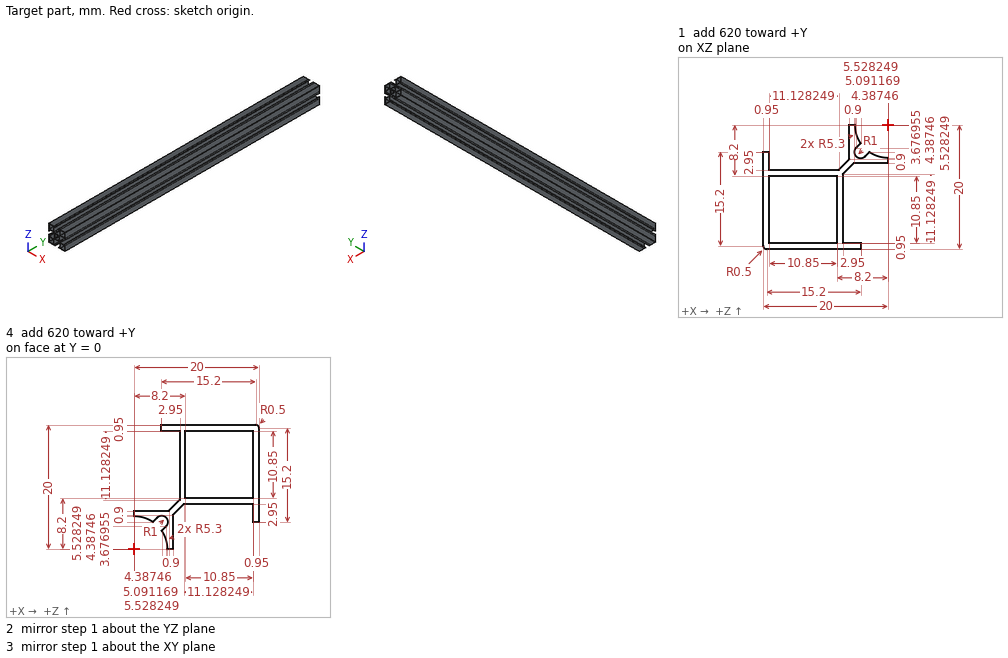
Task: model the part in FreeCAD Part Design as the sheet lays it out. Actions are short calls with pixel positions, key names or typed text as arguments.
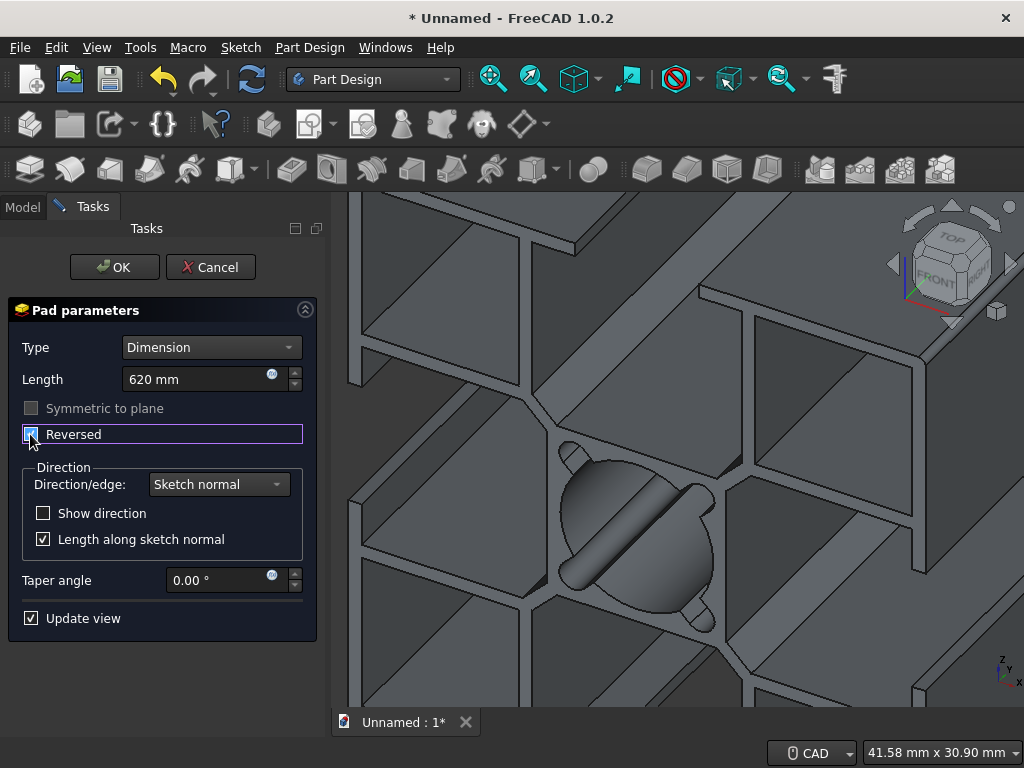
click(115, 267)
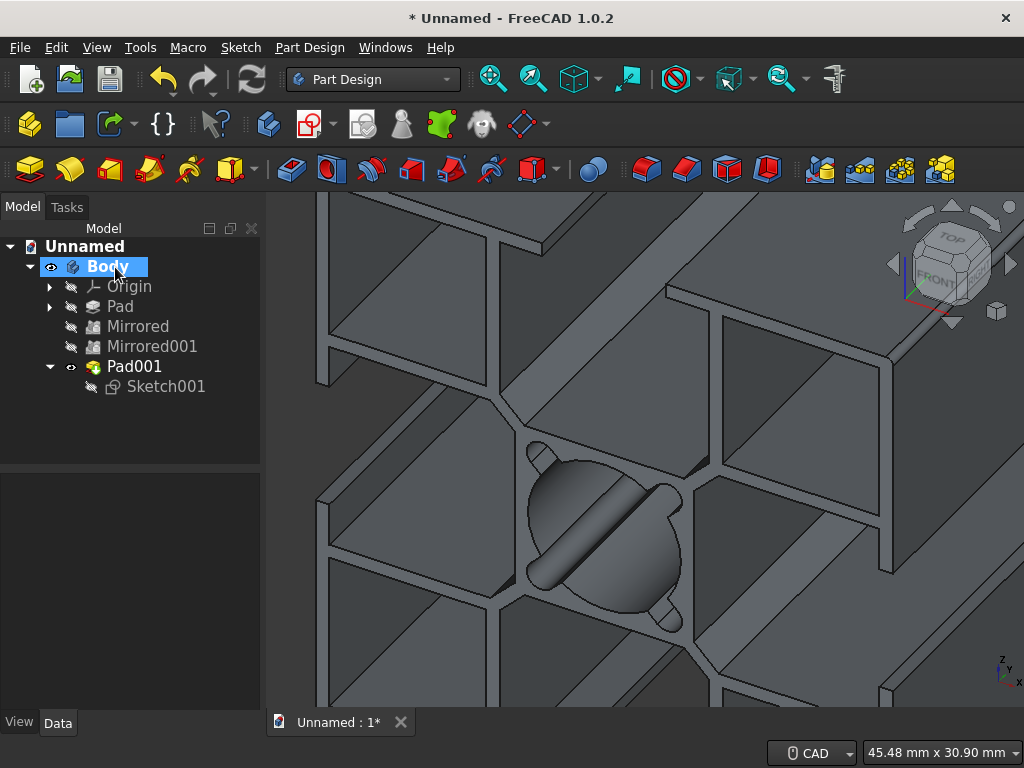
key(0)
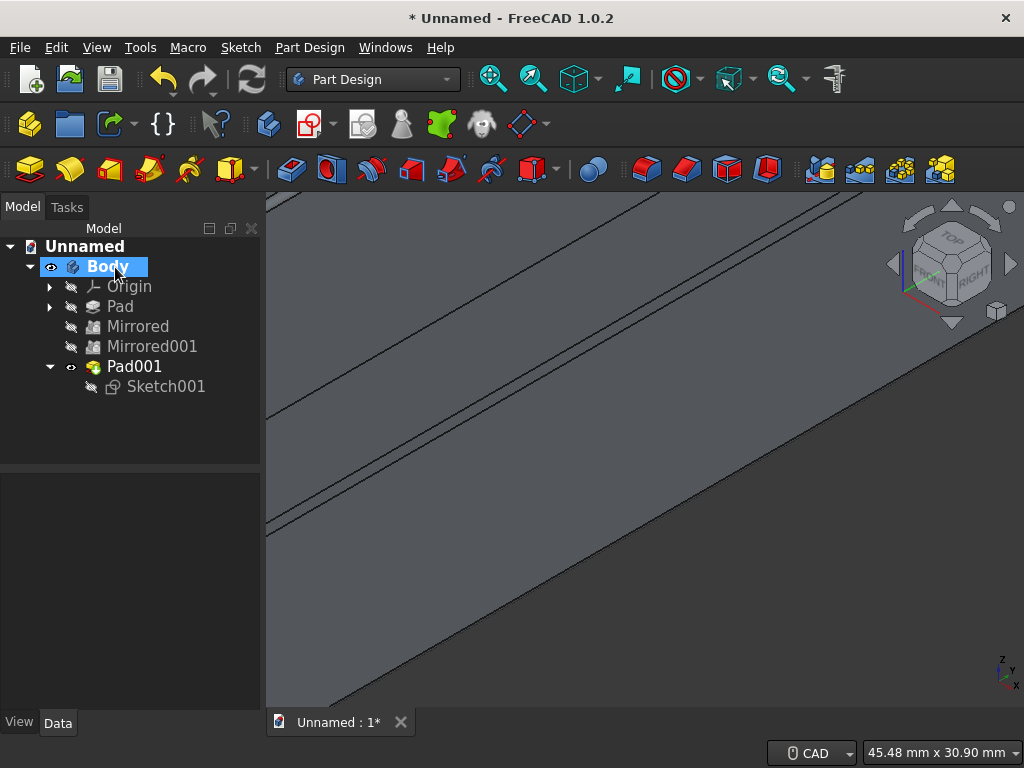
click(494, 80)